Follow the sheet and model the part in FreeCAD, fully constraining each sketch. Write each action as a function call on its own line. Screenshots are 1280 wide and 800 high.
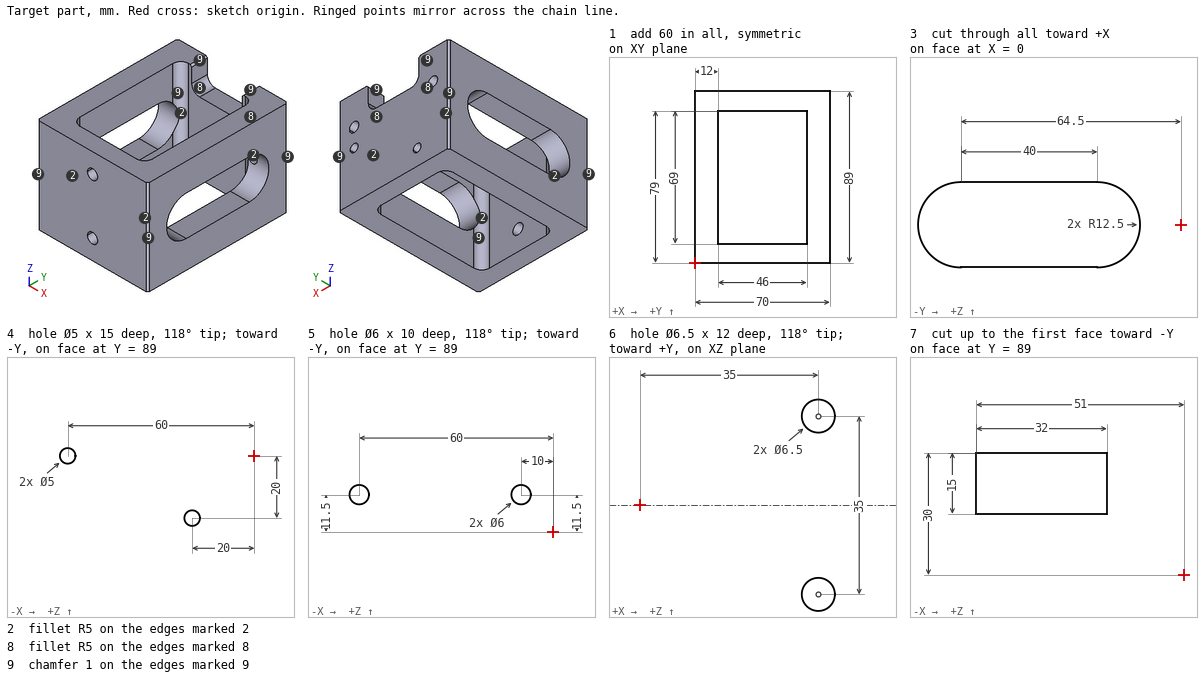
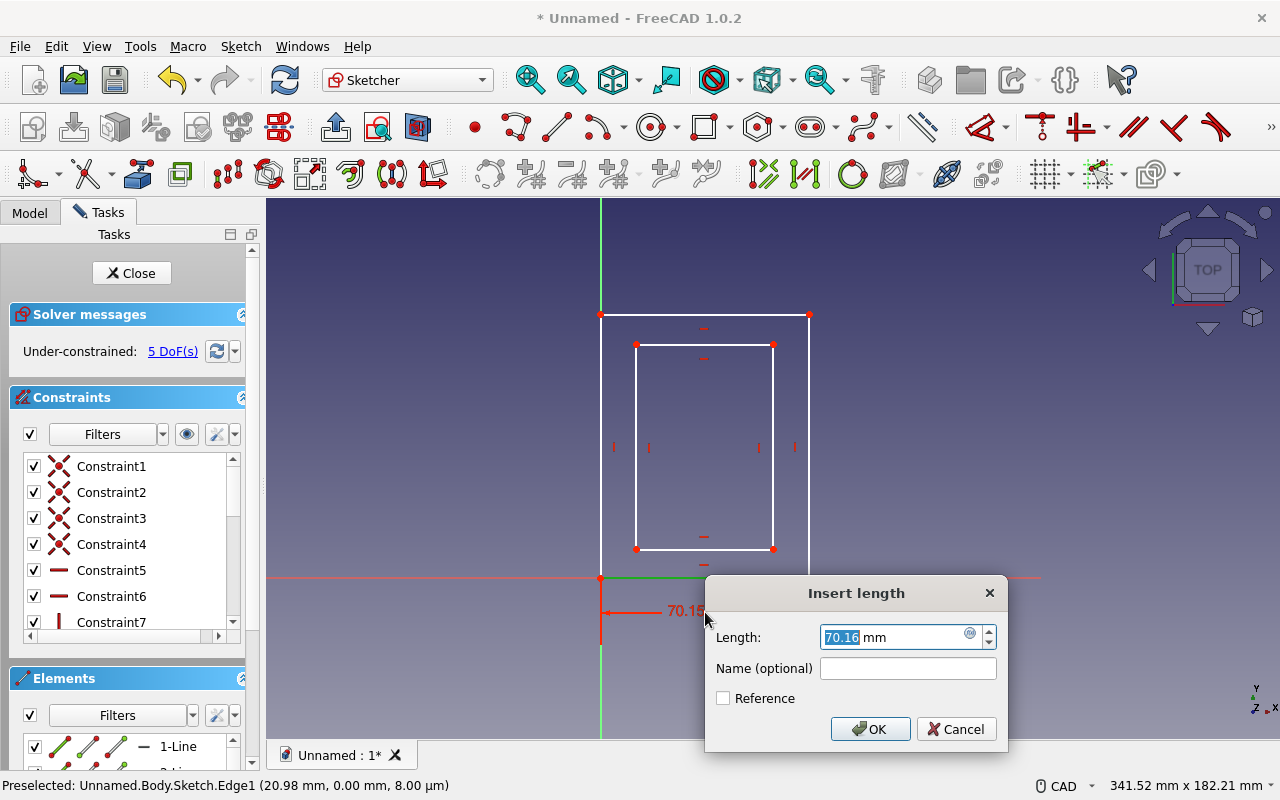
text(70)
key(Return)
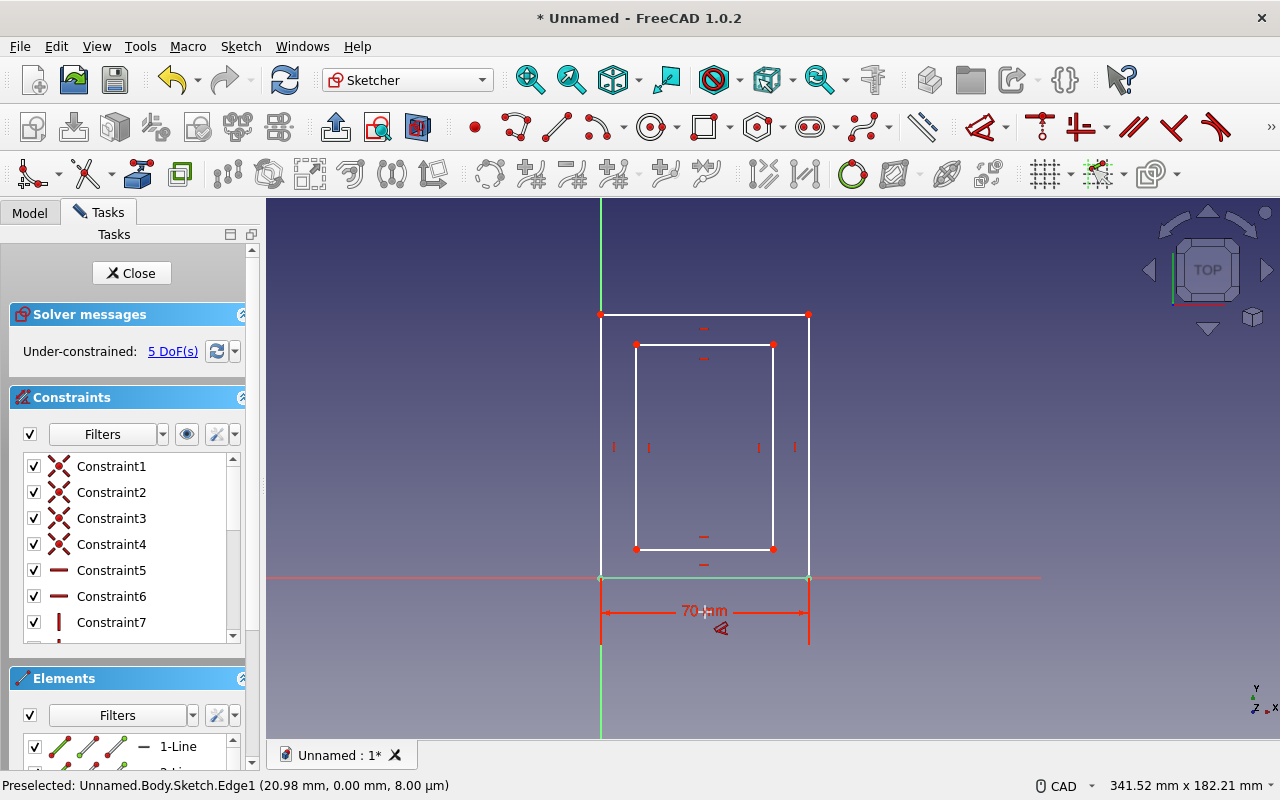
click(809, 499)
click(843, 447)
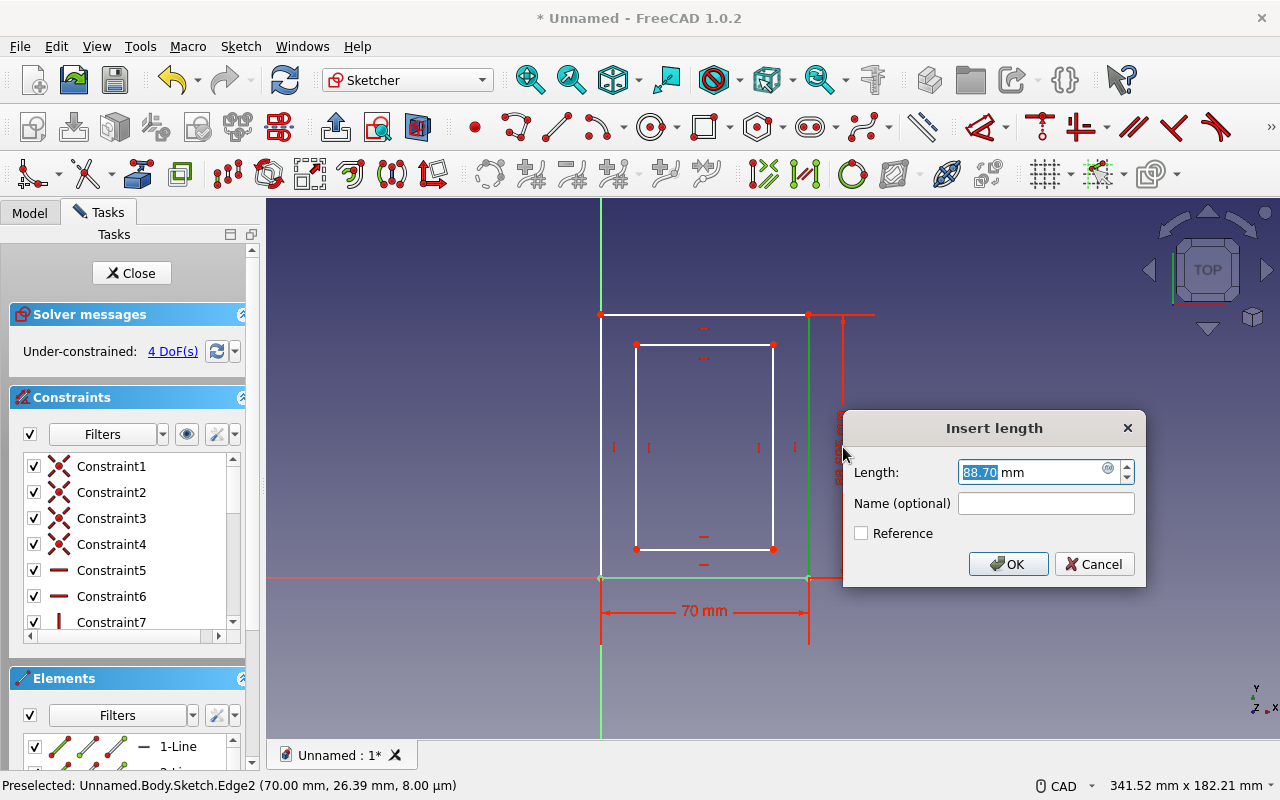
text(89)
key(Return)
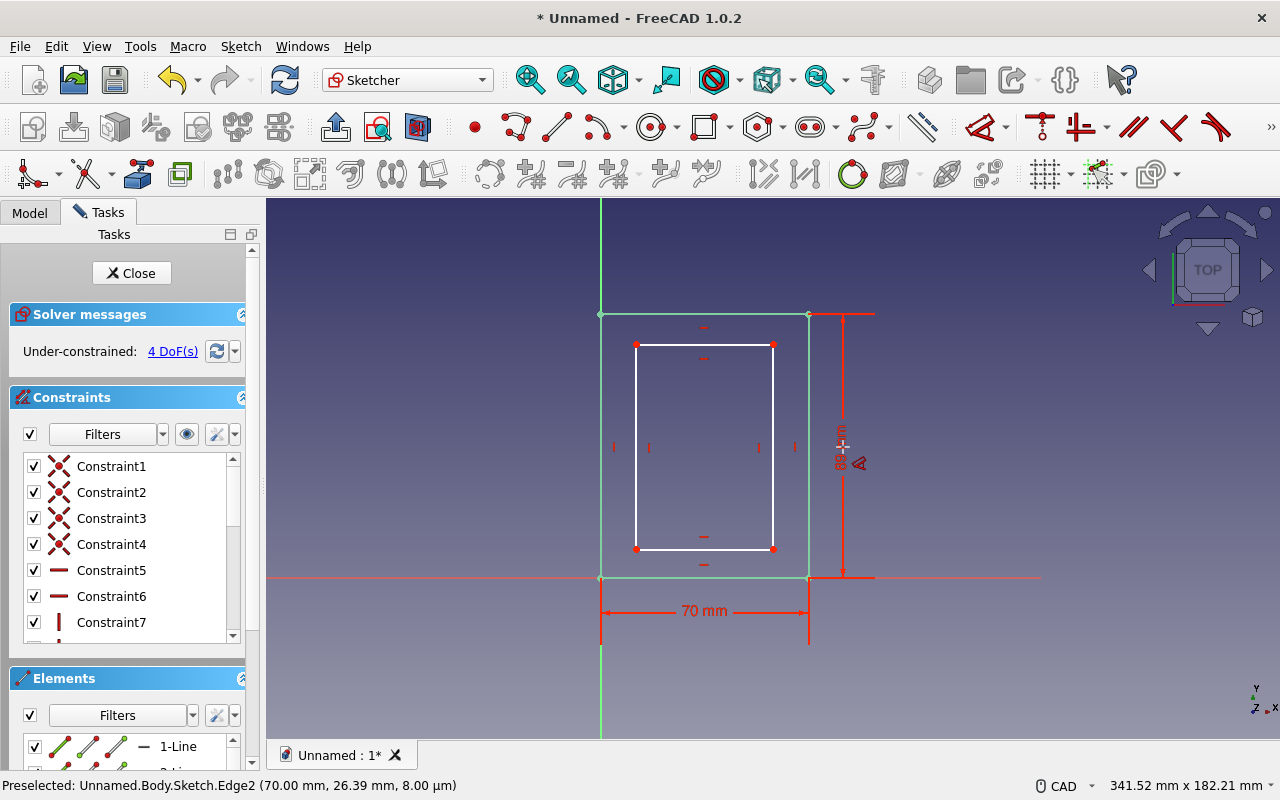
click(636, 407)
click(670, 448)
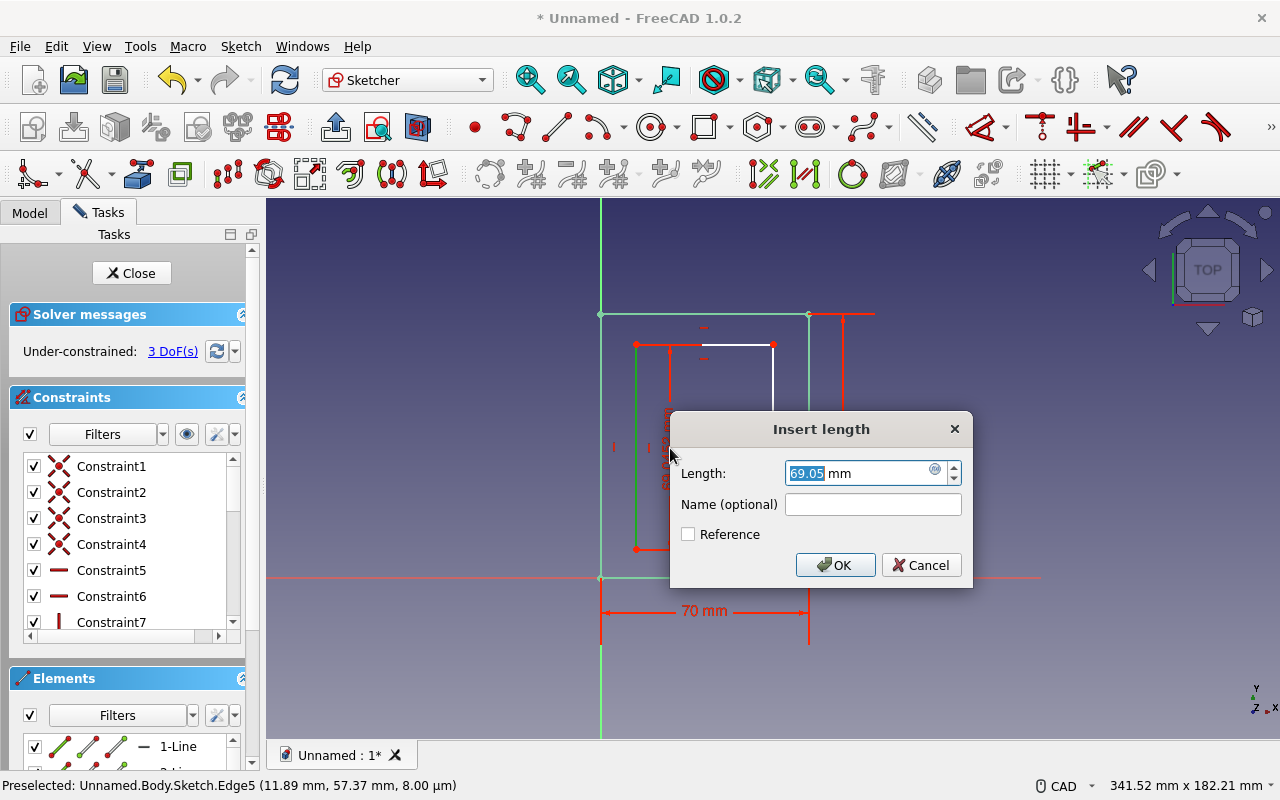
text(69)
key(Return)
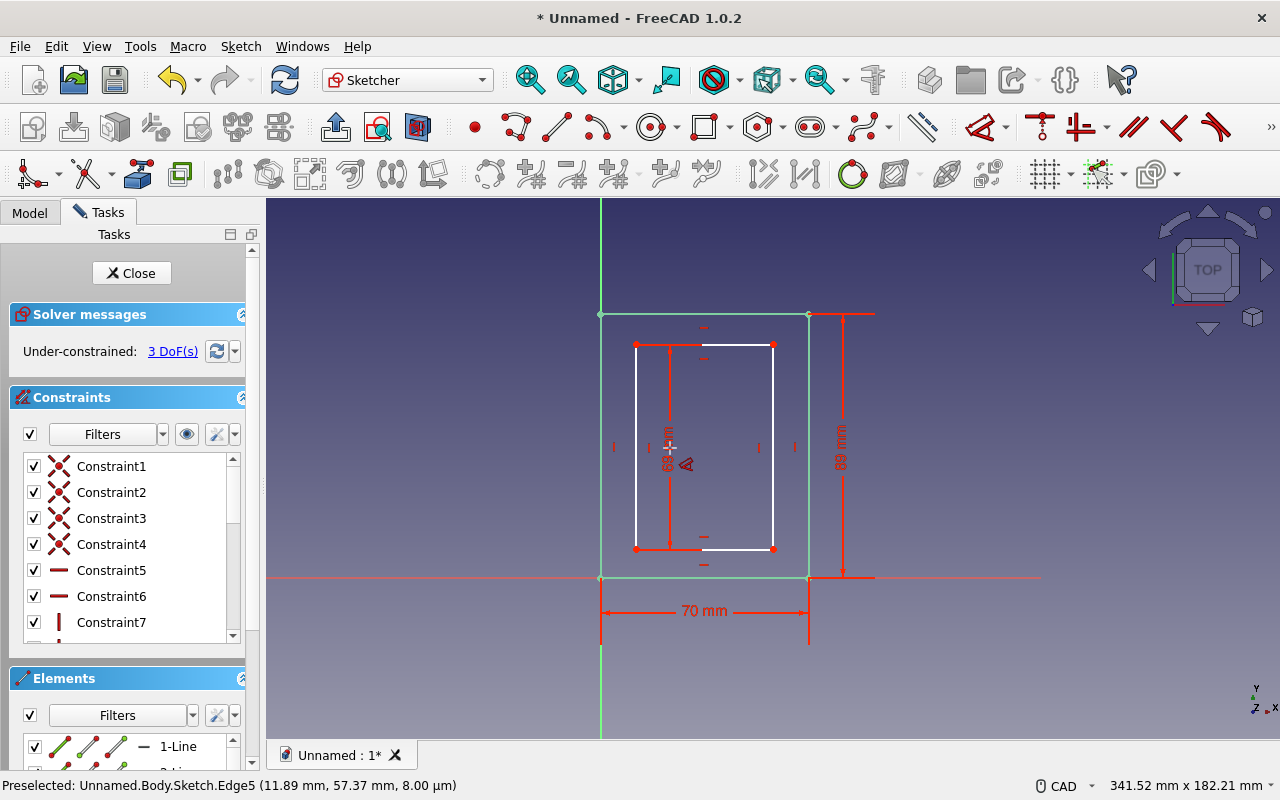
click(677, 550)
click(705, 516)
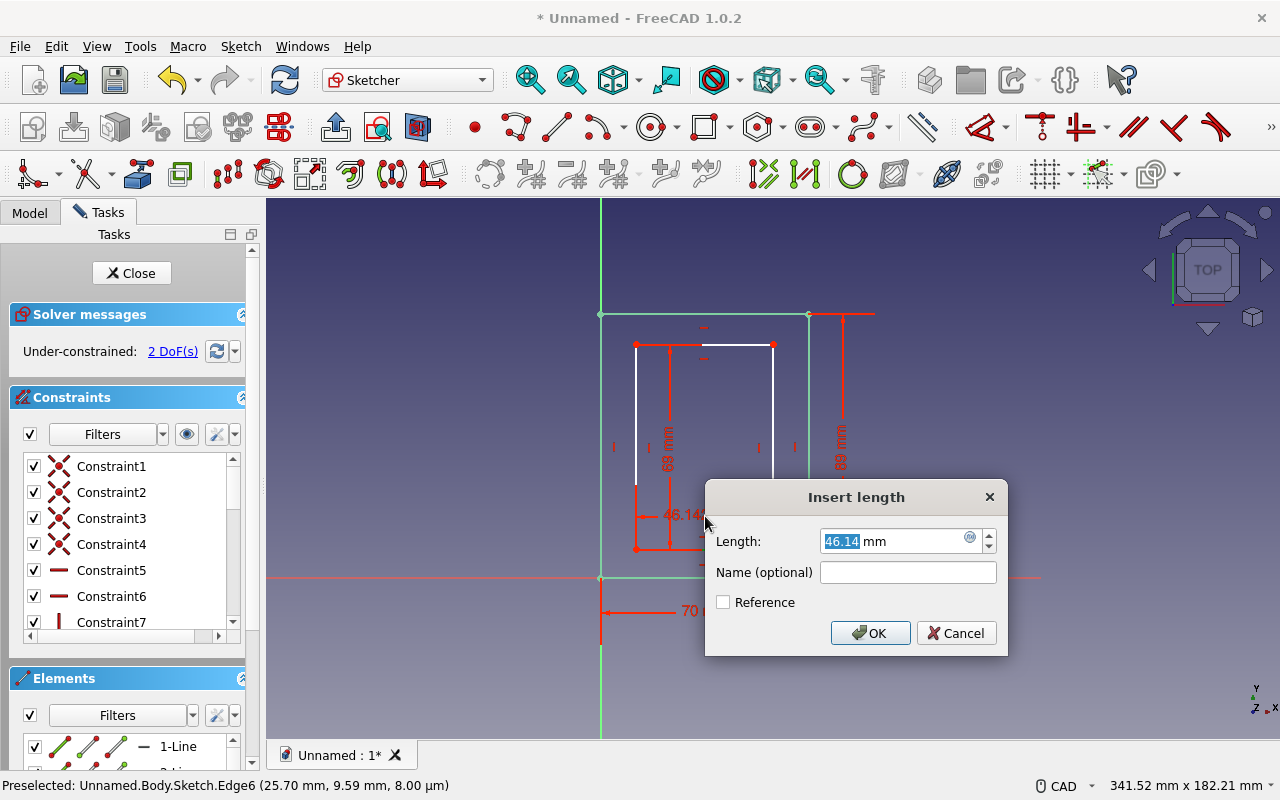
text(46)
key(Return)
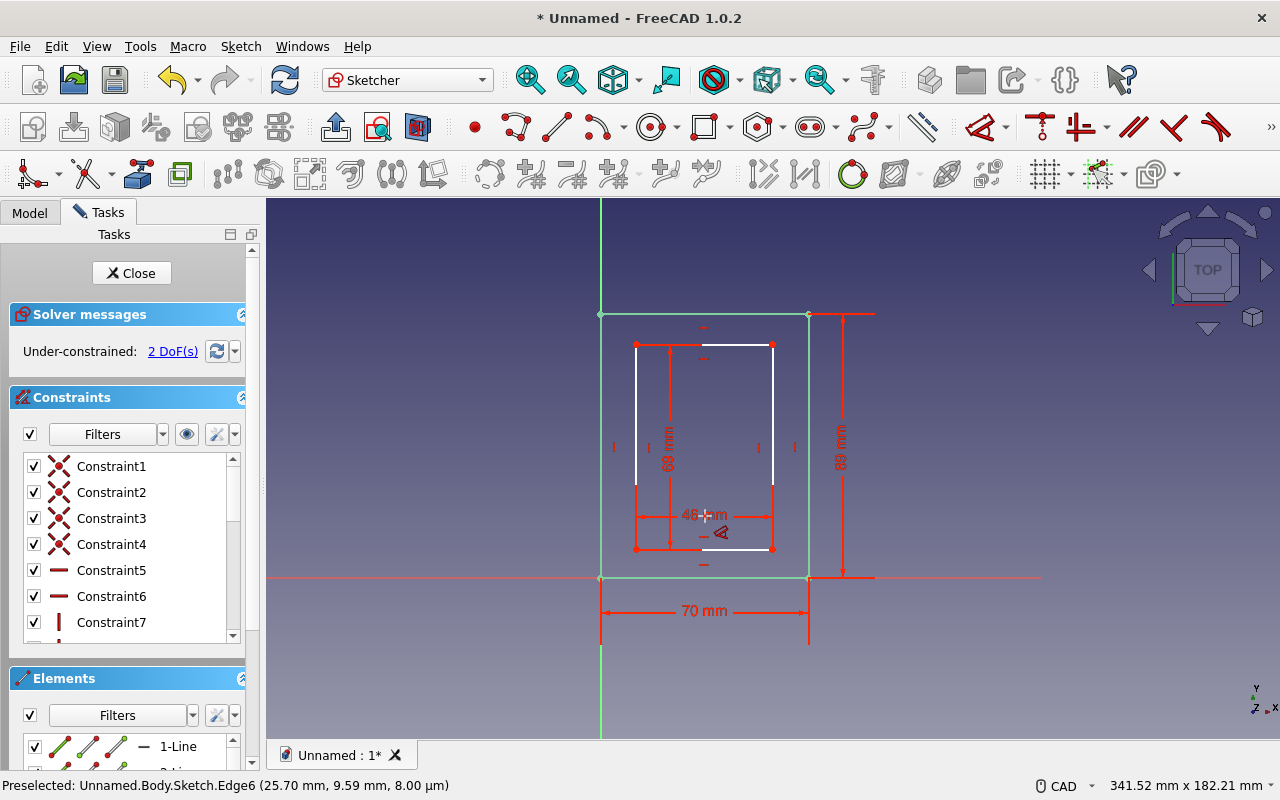
click(636, 345)
click(618, 612)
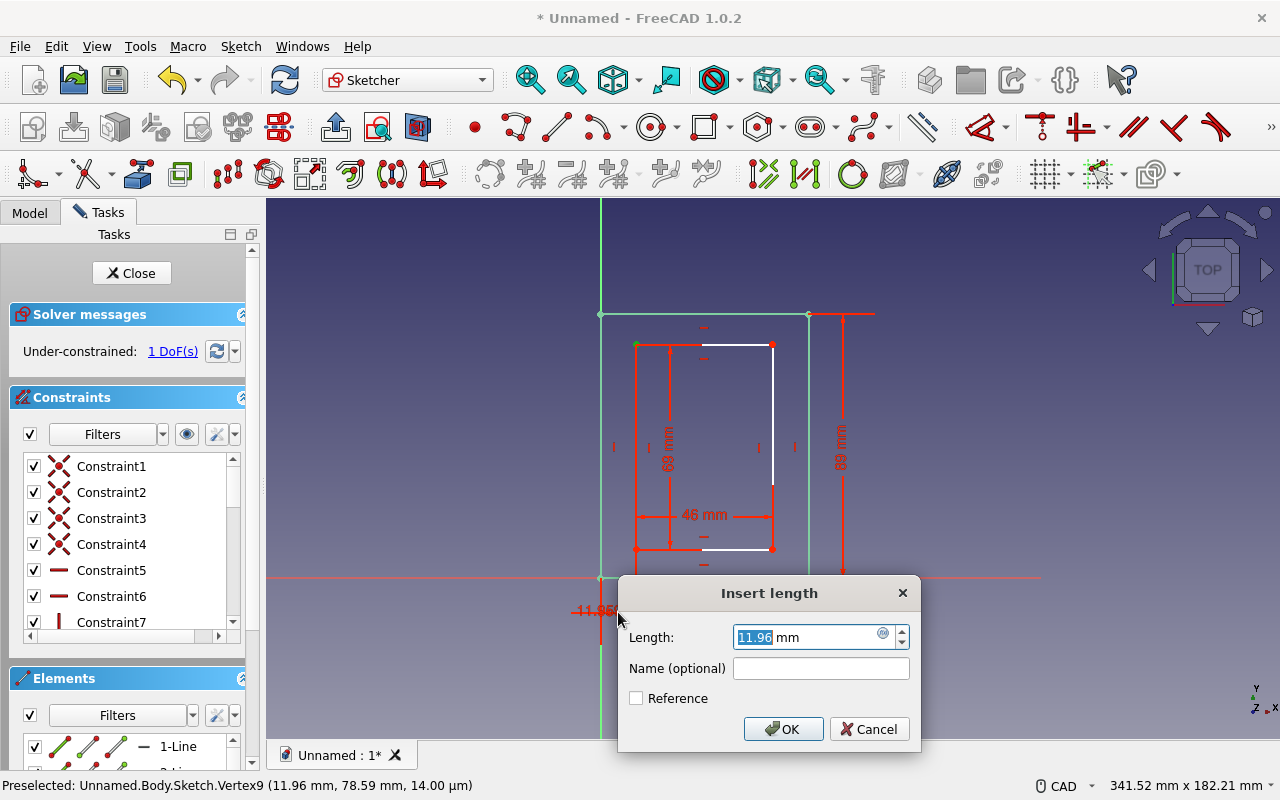
text(12)
key(Return)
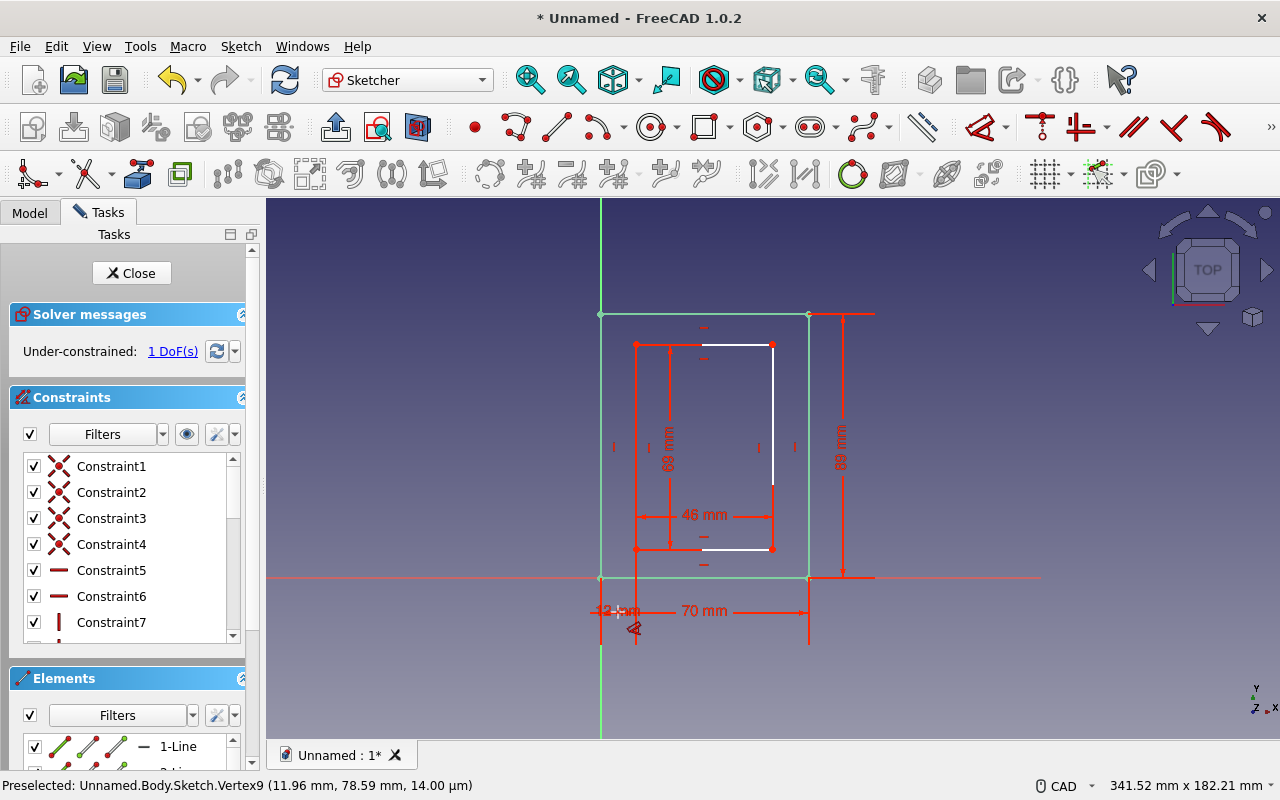
click(636, 345)
click(567, 462)